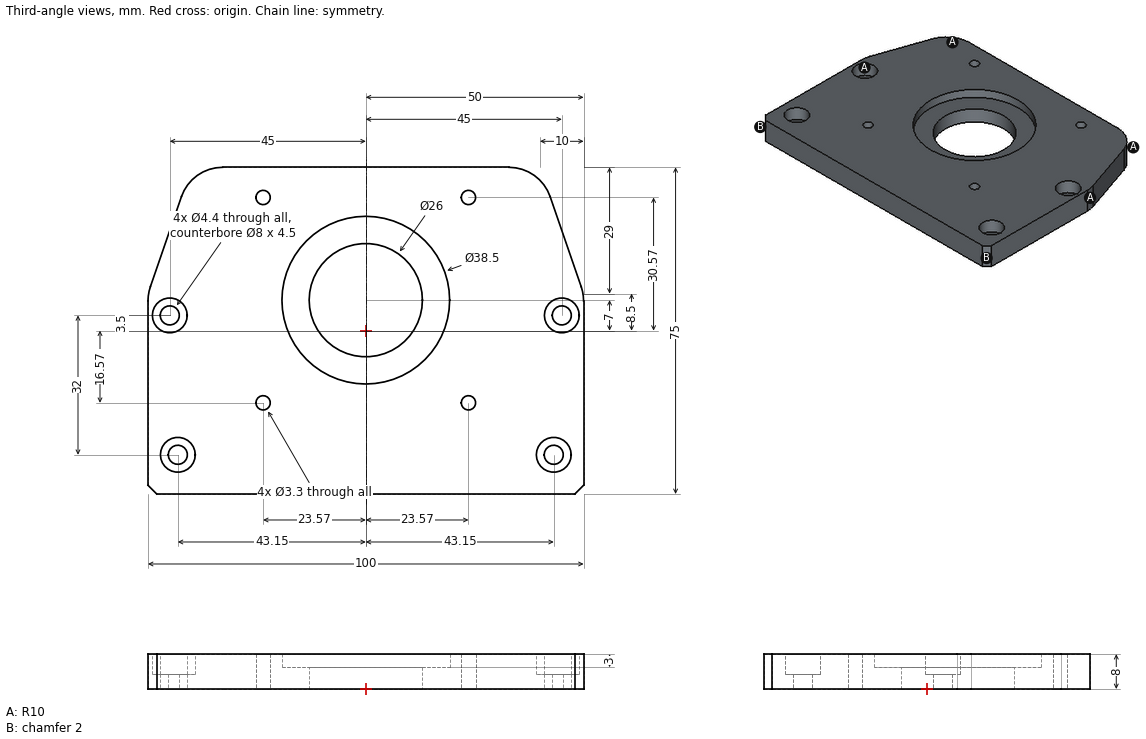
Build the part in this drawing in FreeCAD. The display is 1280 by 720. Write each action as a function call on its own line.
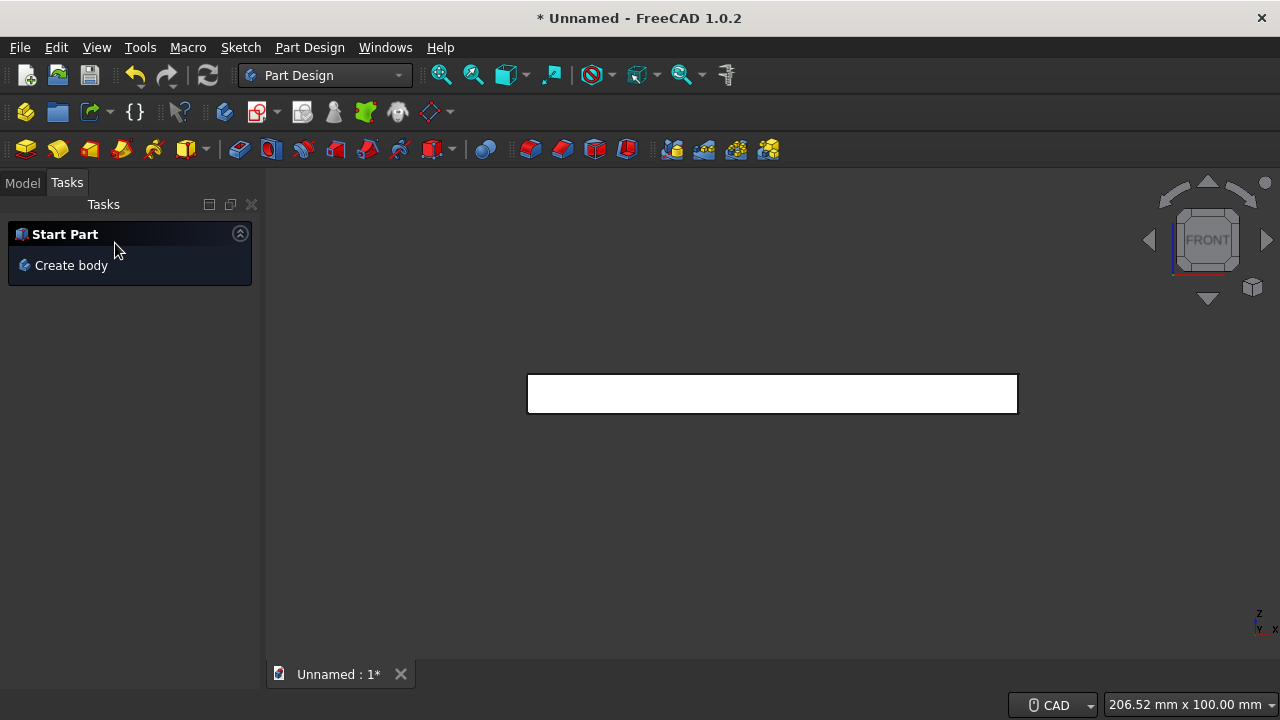
key(3)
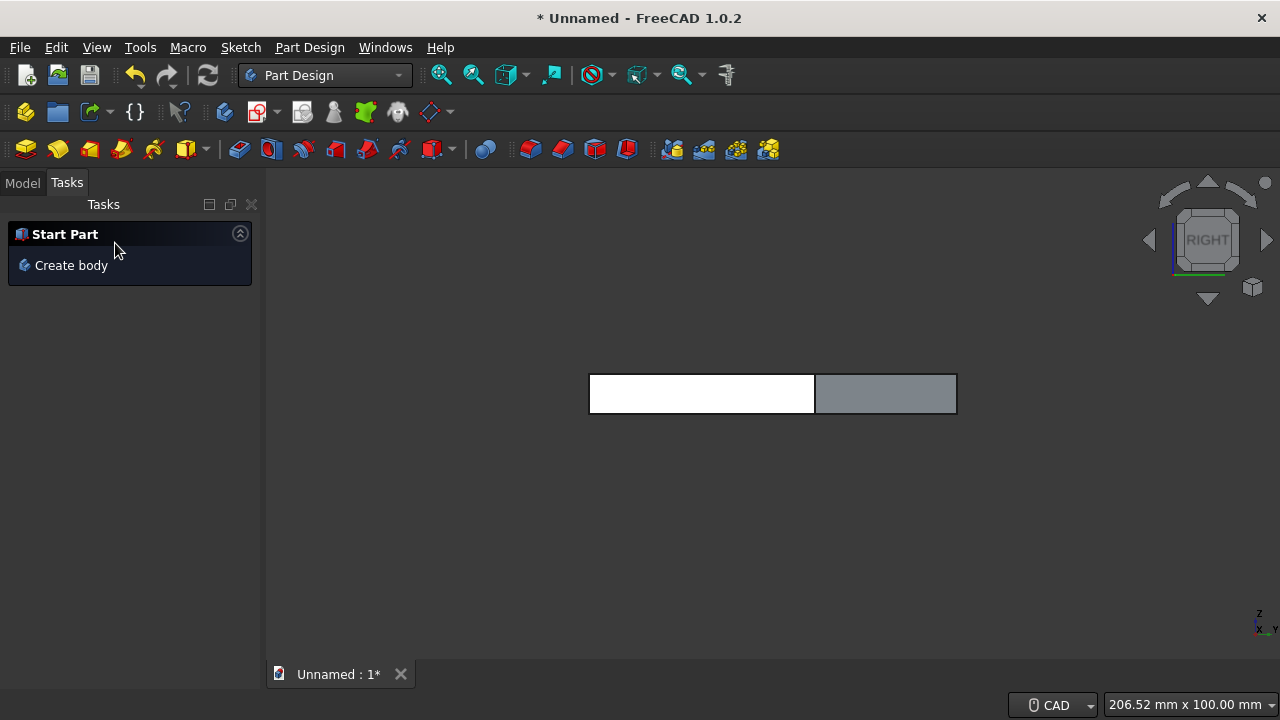
click(442, 76)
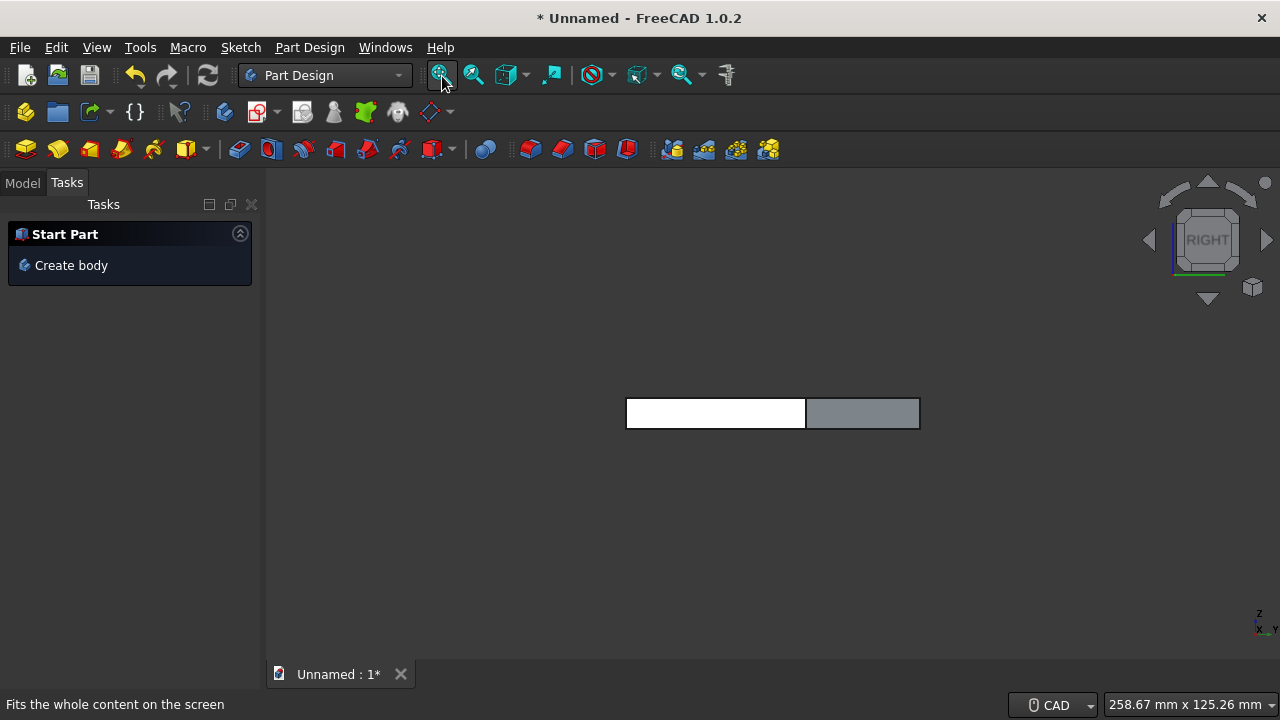
click(806, 412)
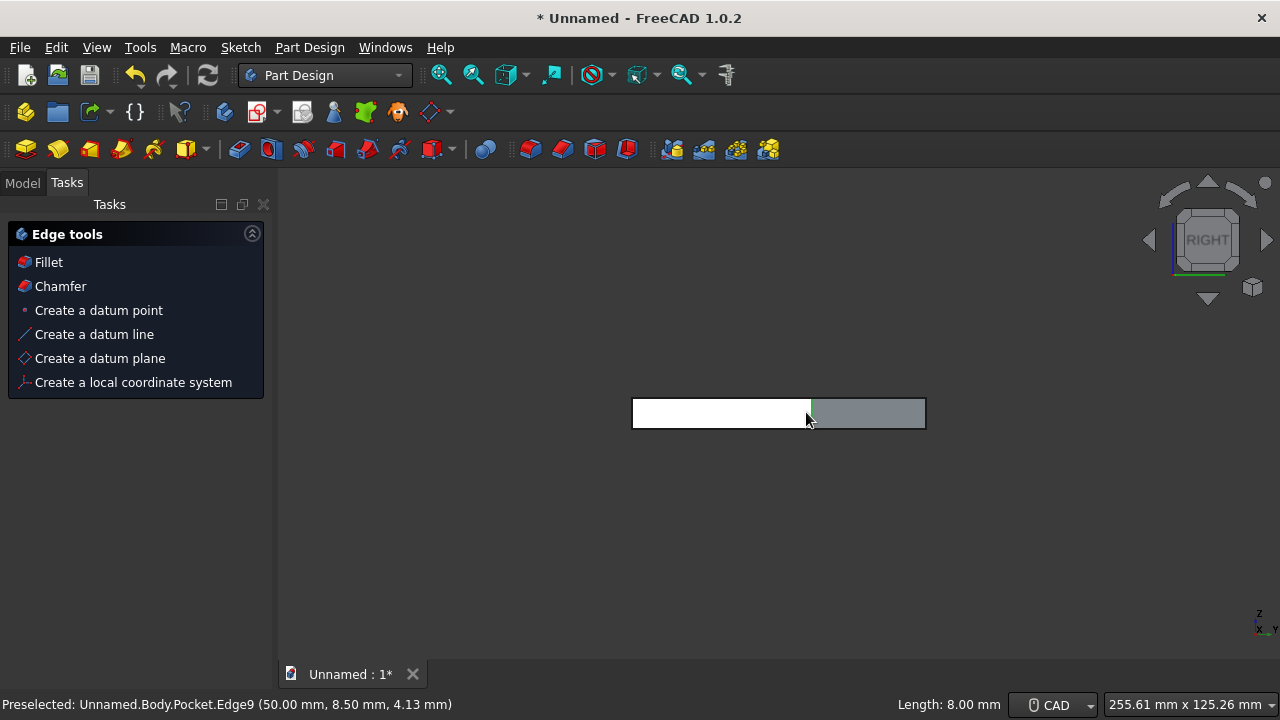
key(5)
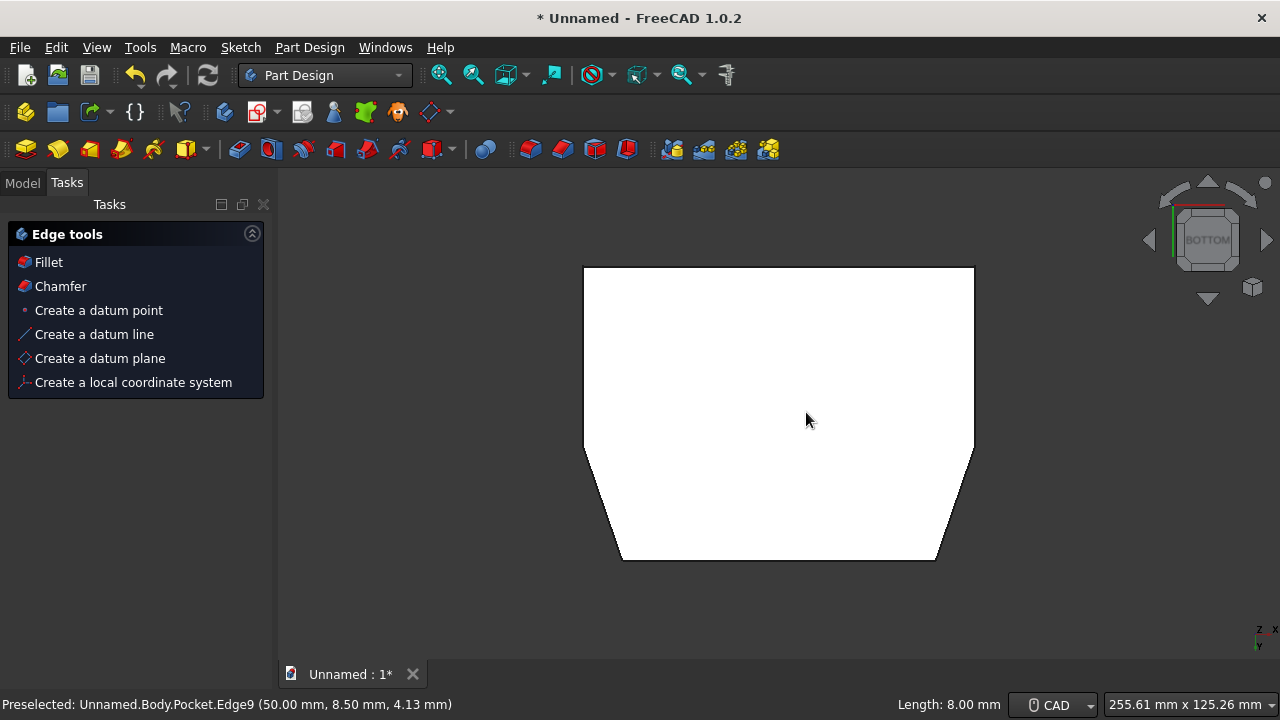
key(4)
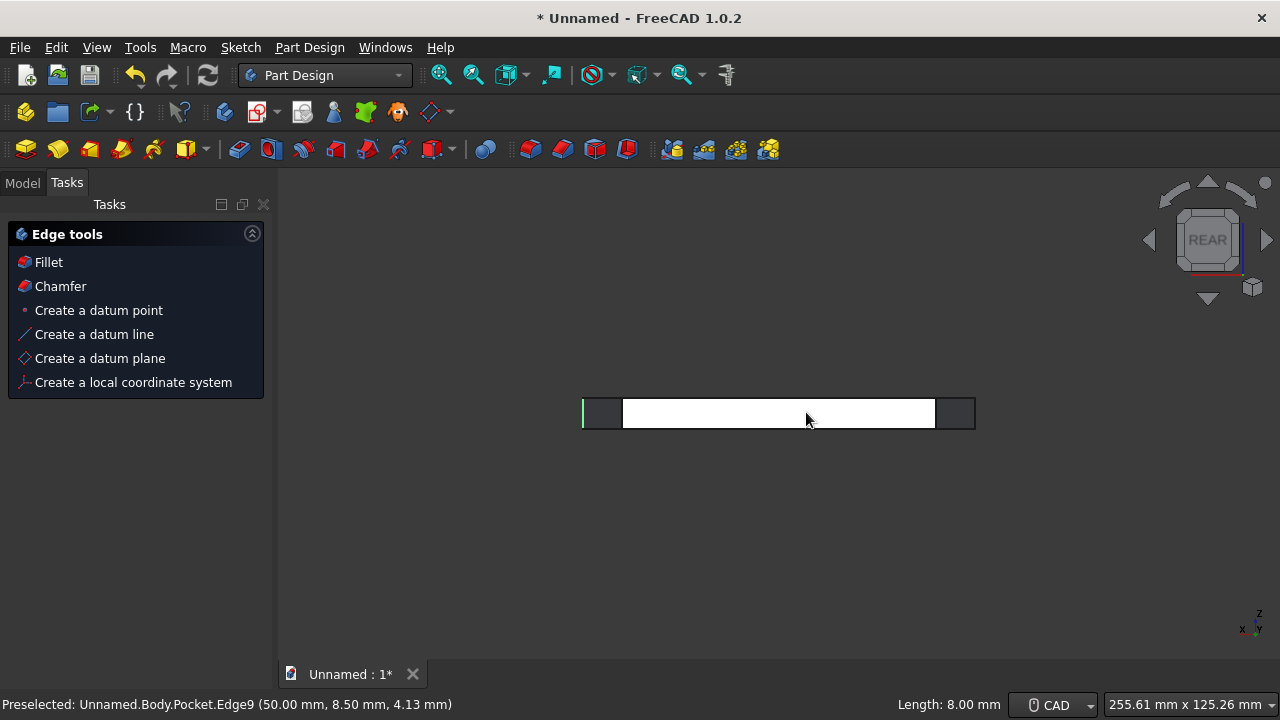
click(442, 76)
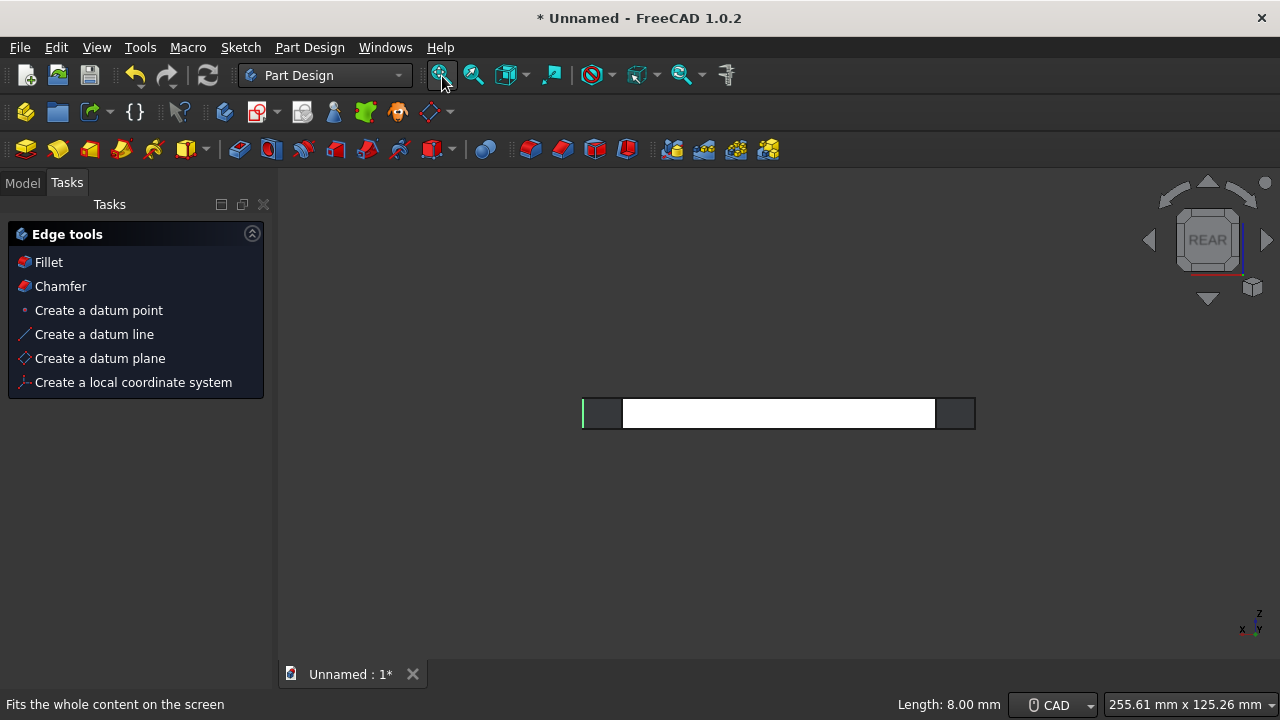
click(622, 413, ctrl)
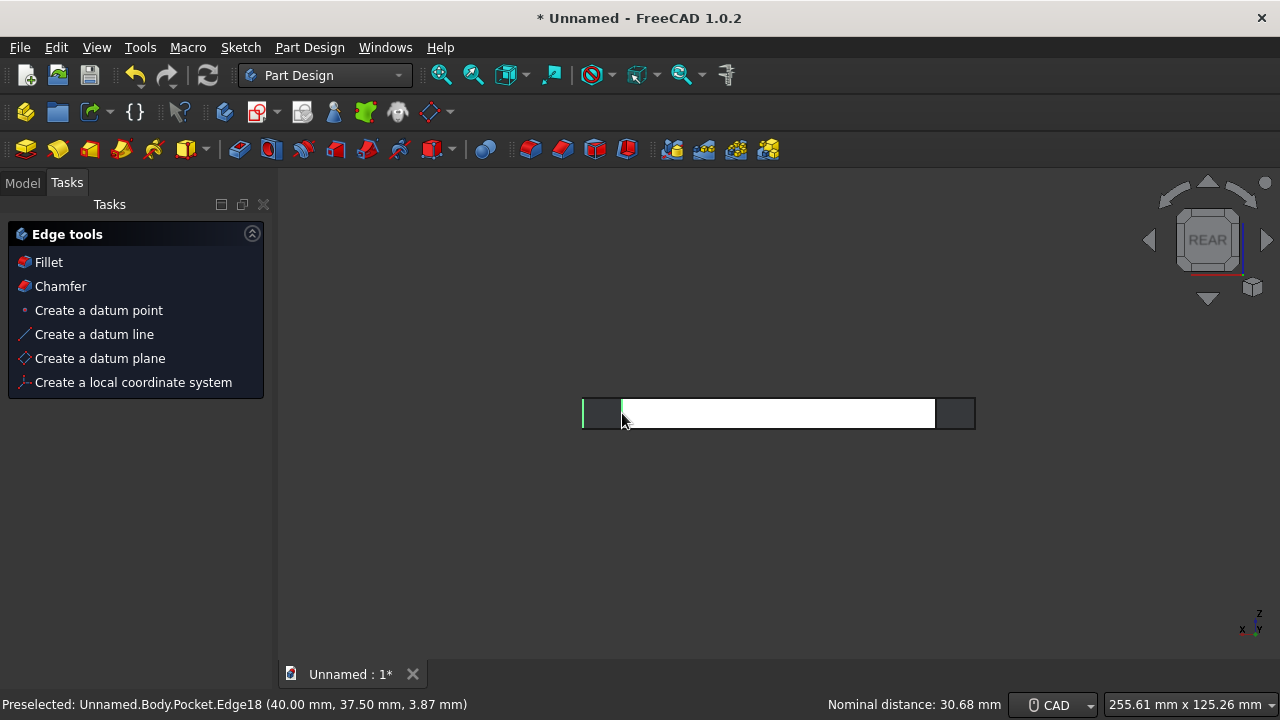
click(936, 413, ctrl)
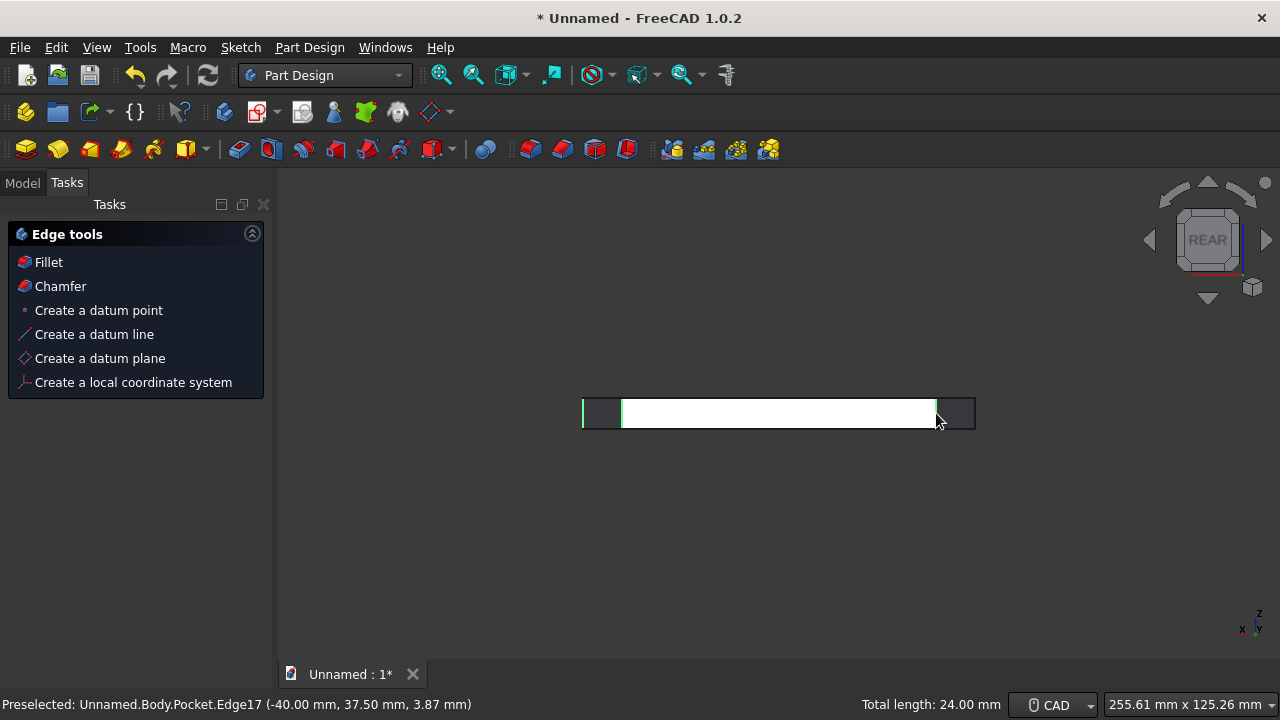
key(6)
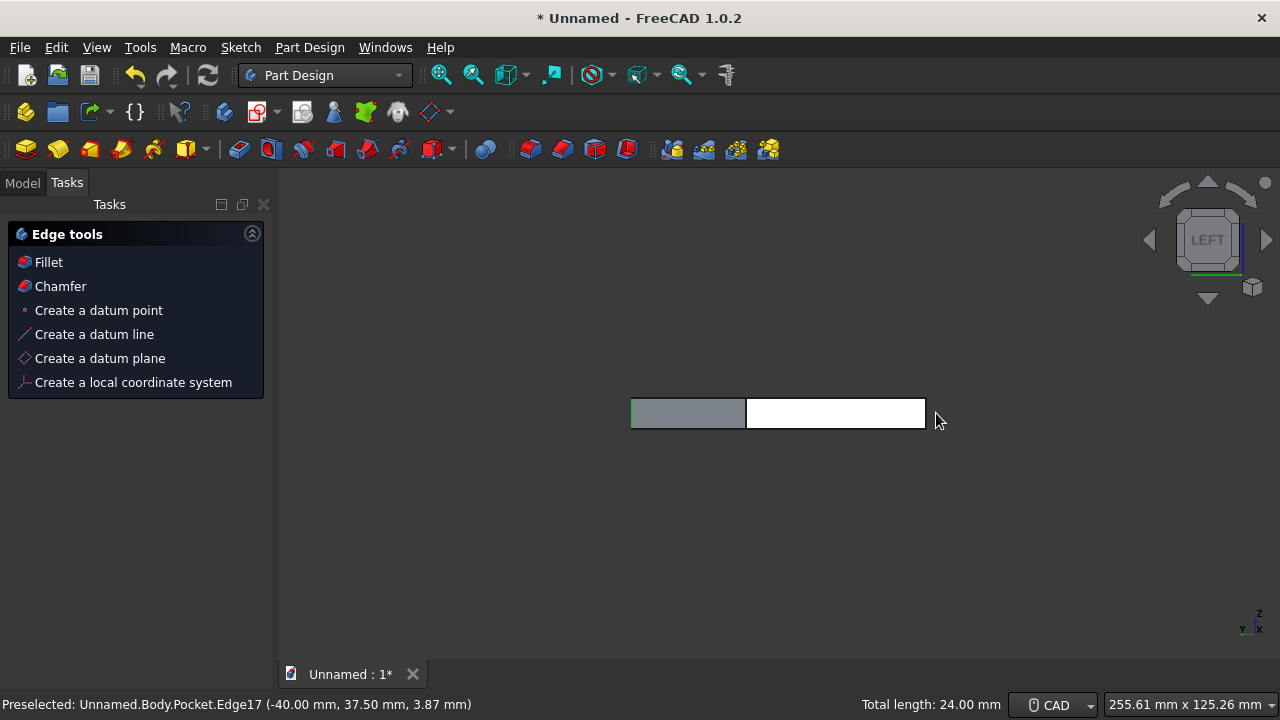
key(v)
key(f)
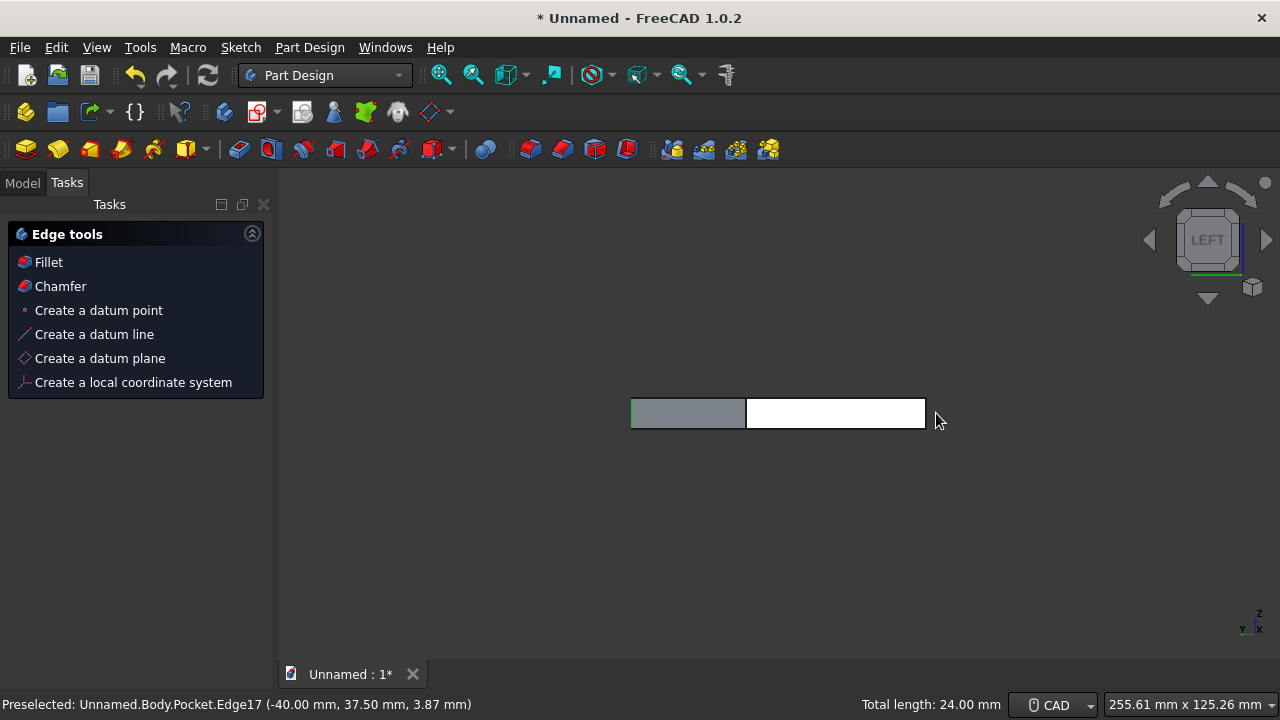
click(746, 412, ctrl)